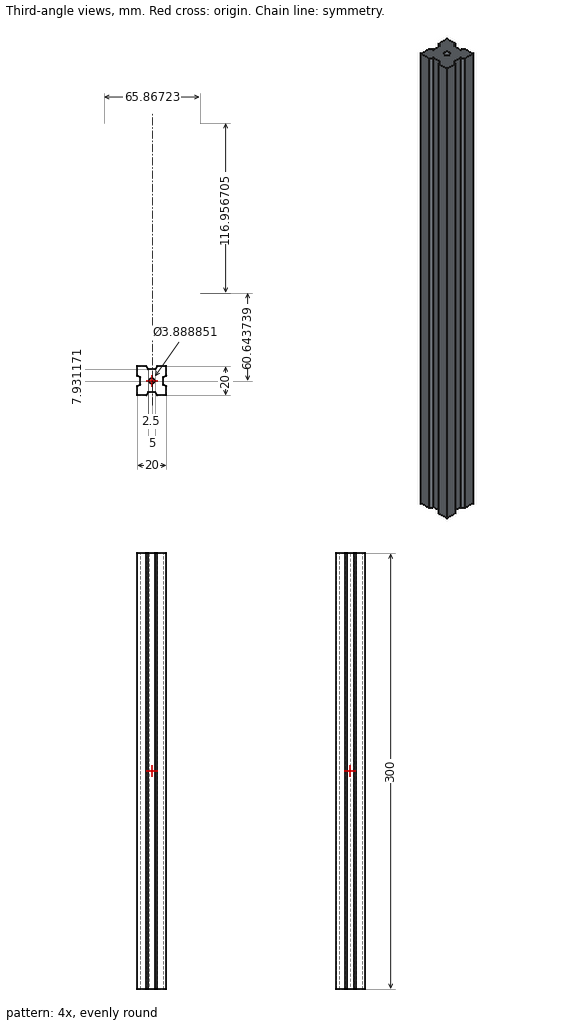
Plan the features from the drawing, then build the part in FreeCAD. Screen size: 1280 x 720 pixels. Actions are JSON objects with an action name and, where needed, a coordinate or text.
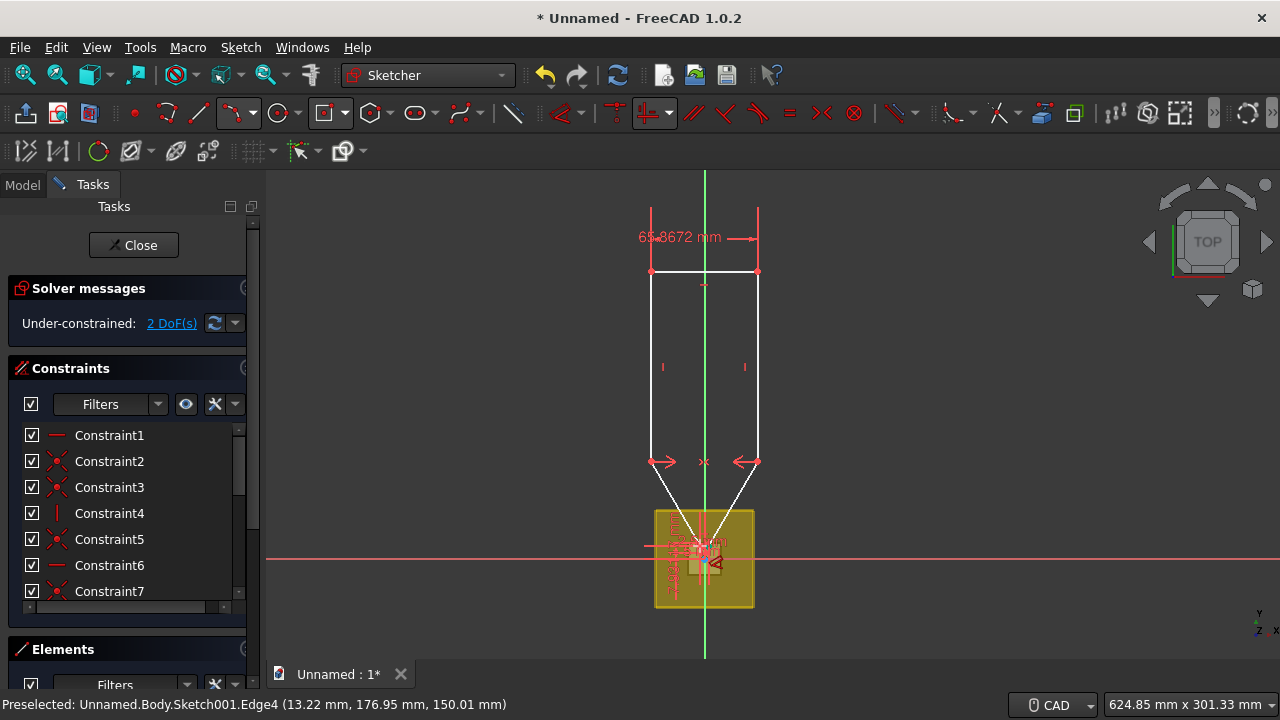
{"action": "left_click", "coordinate": [758, 405]}
{"action": "left_click", "coordinate": [792, 367]}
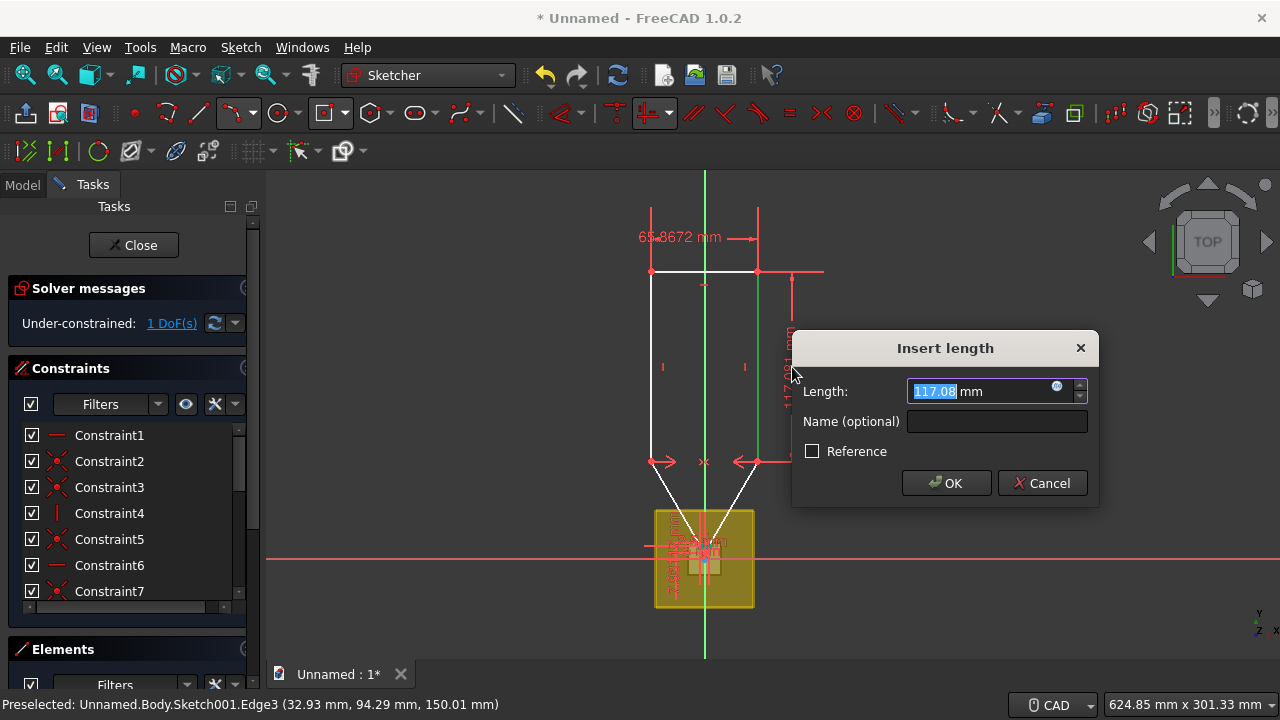
{"action": "type", "text": "116.956705"}
{"action": "key", "text": "Return"}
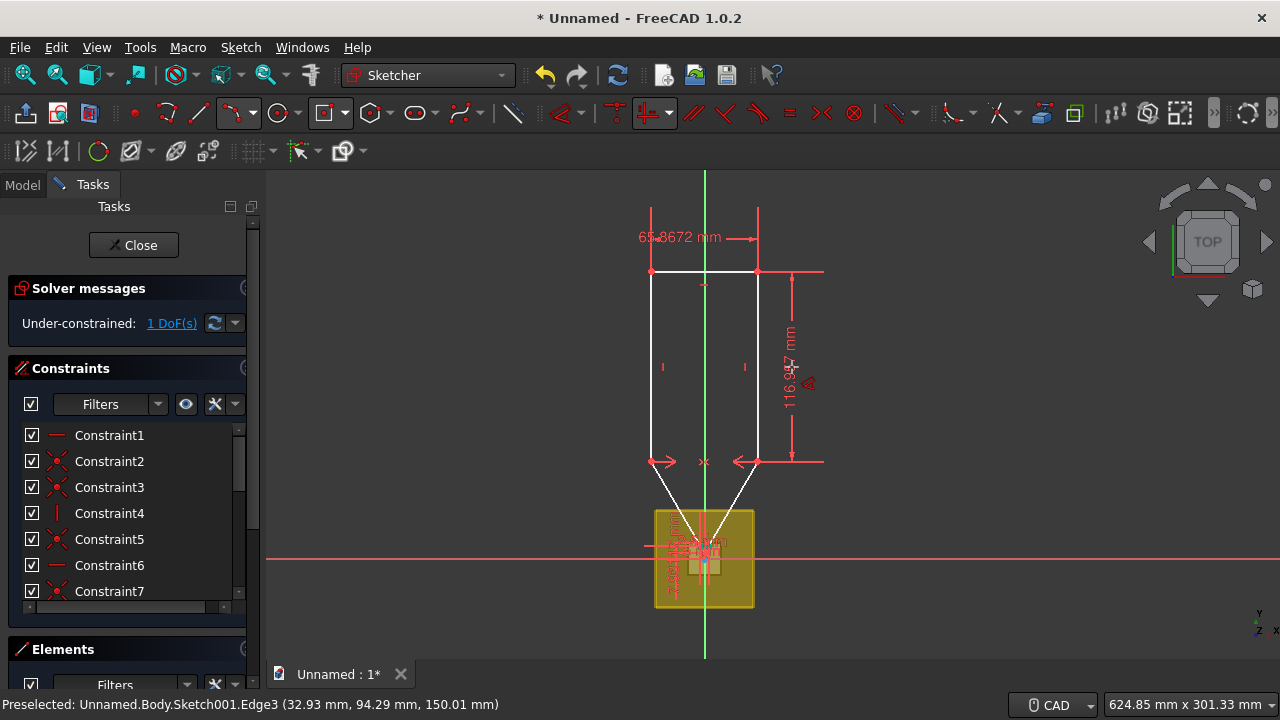
{"action": "left_click", "coordinate": [758, 462]}
{"action": "left_click", "coordinate": [792, 510]}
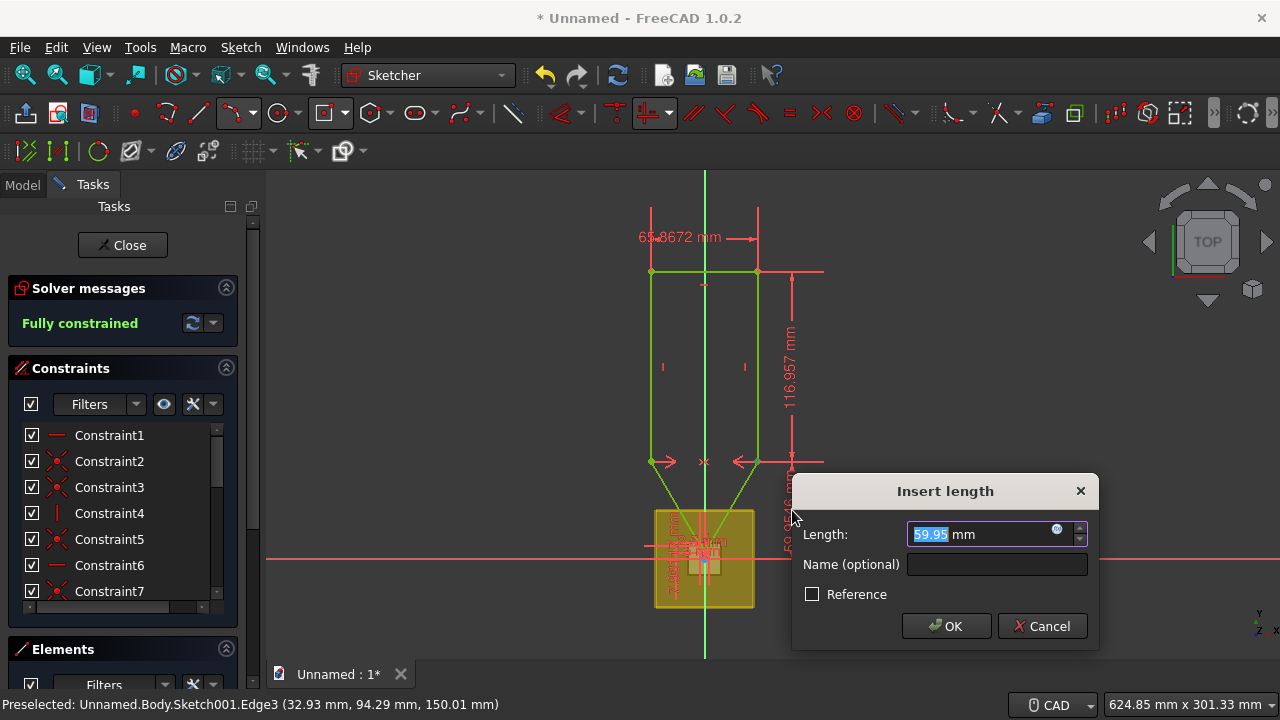
{"action": "type", "text": "60.643739"}
{"action": "key", "text": "Return"}
{"action": "key", "text": "Escape"}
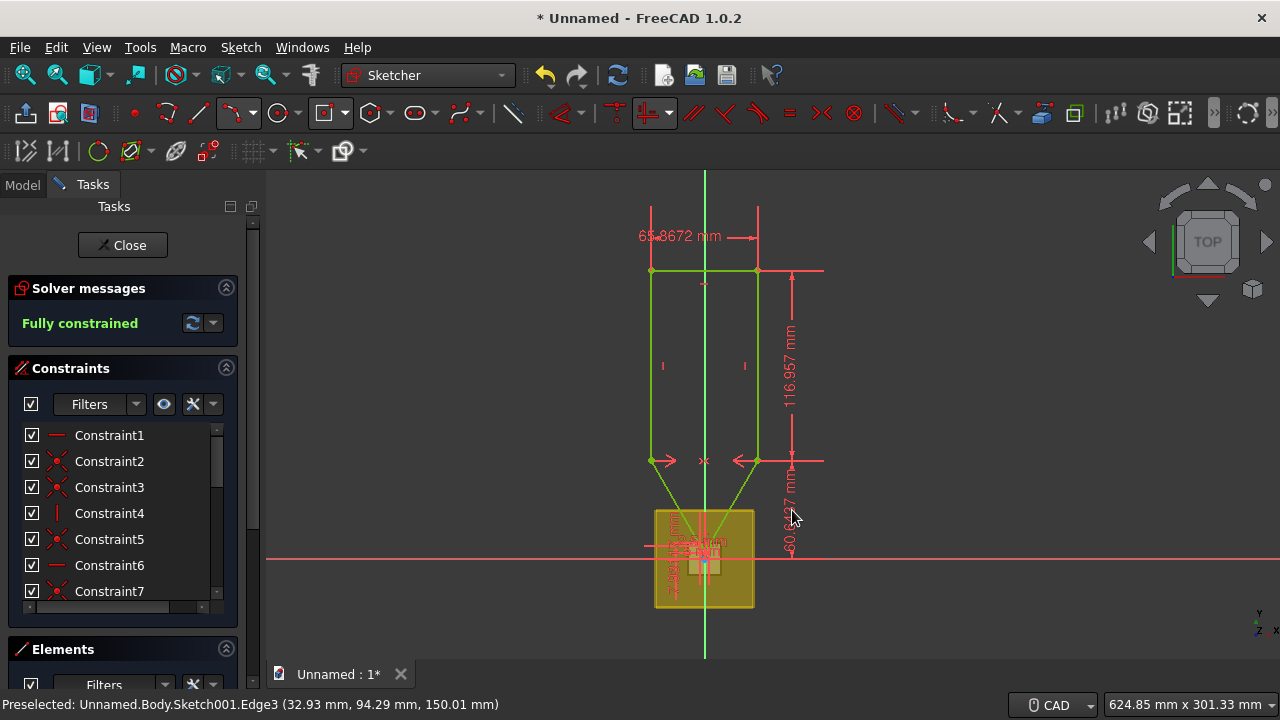
{"action": "left_click", "coordinate": [123, 245]}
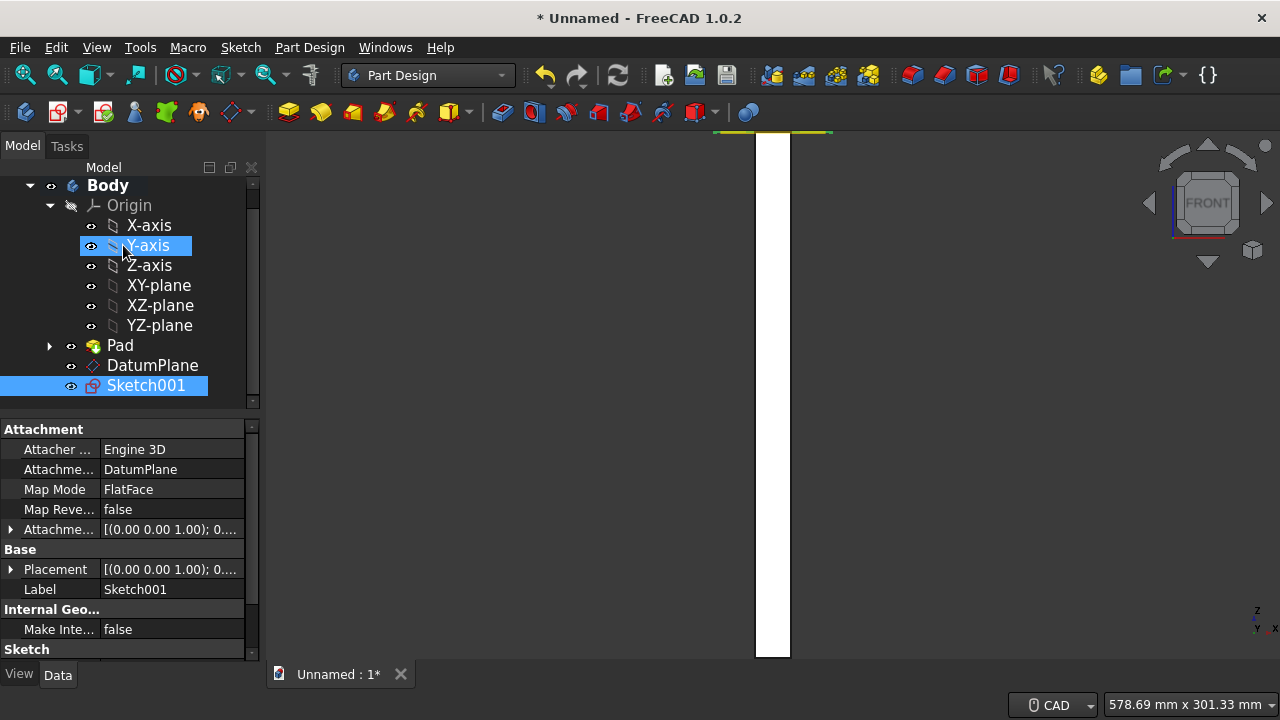
{"action": "left_click", "coordinate": [504, 112]}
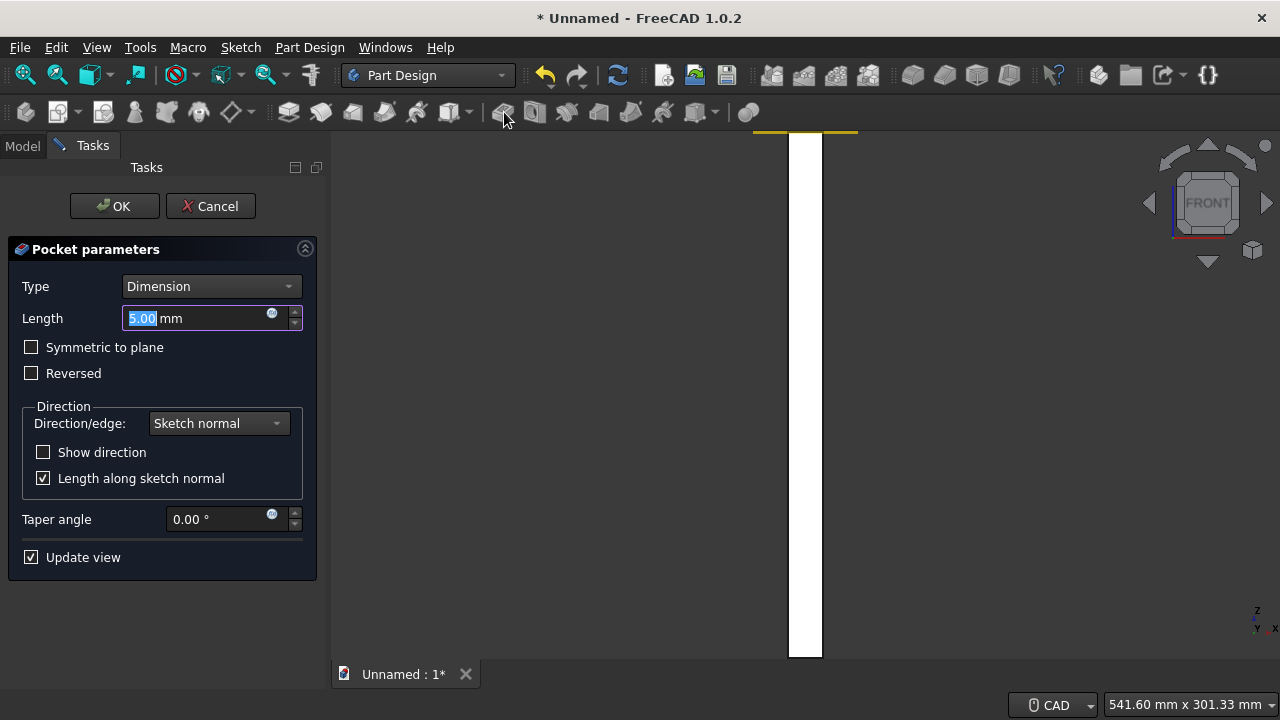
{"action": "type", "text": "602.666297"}
{"action": "key", "text": "Tab"}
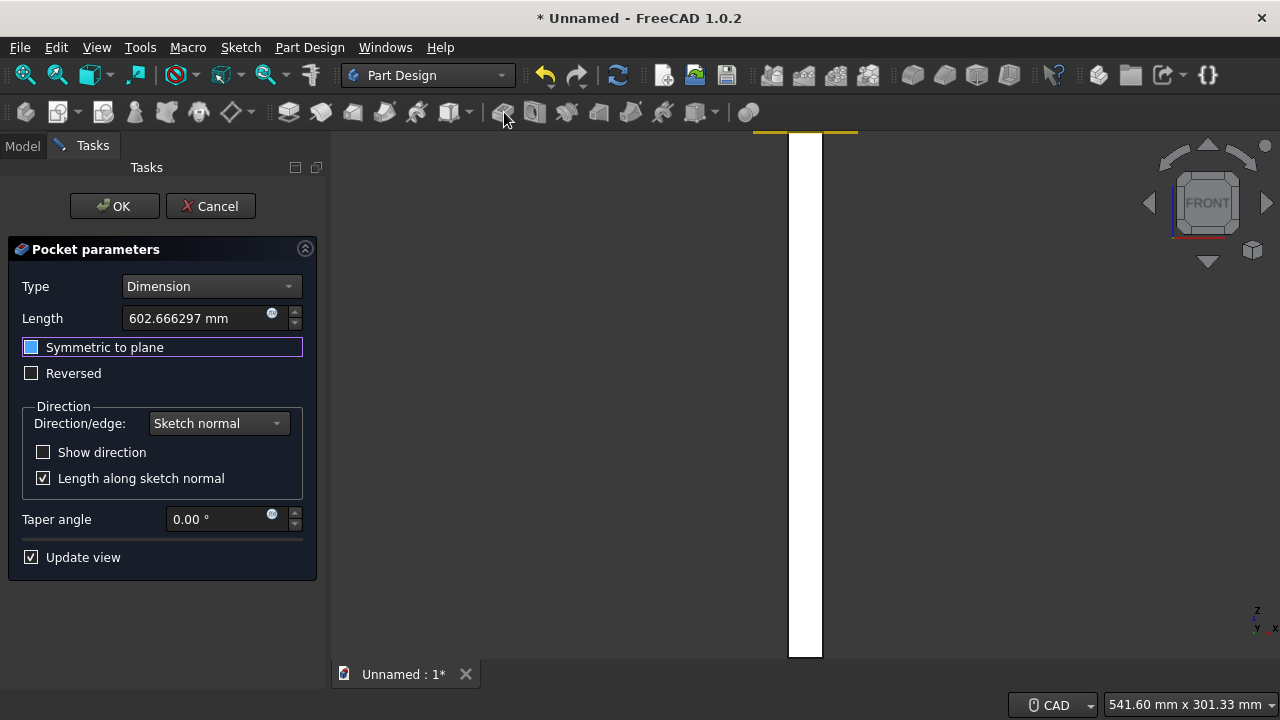
{"action": "left_click", "coordinate": [30, 347]}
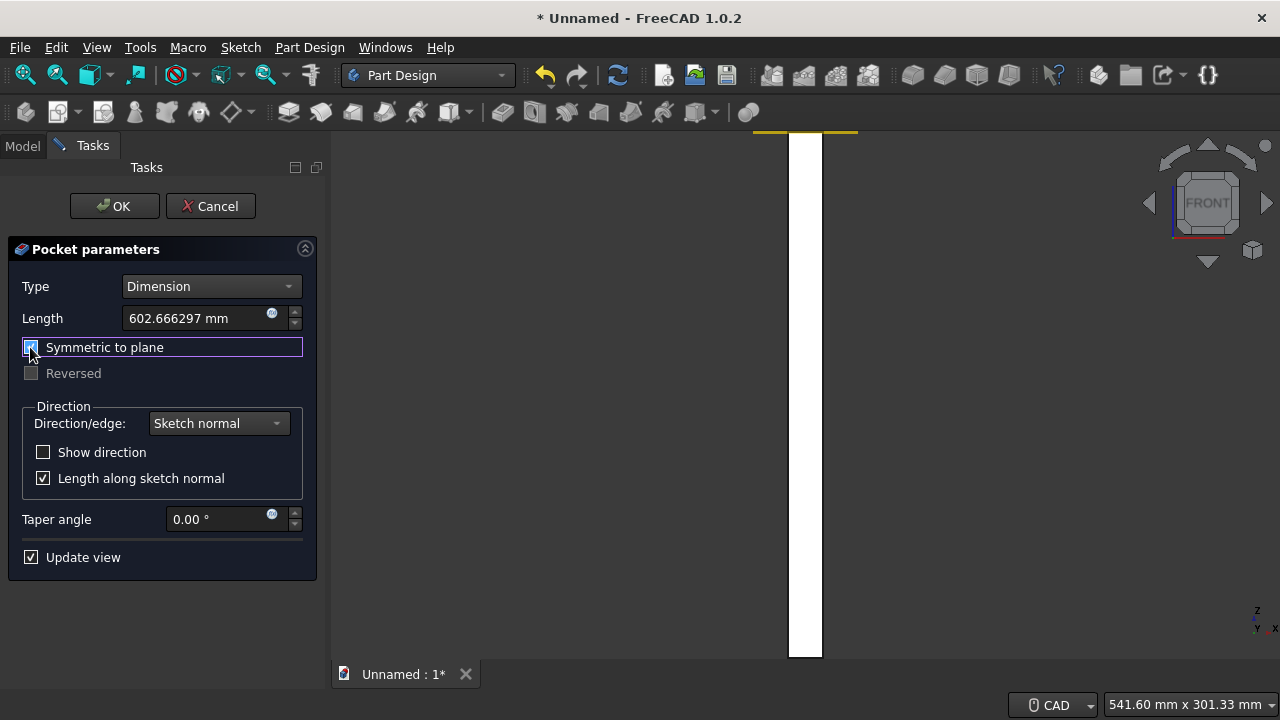
{"action": "left_click", "coordinate": [115, 206]}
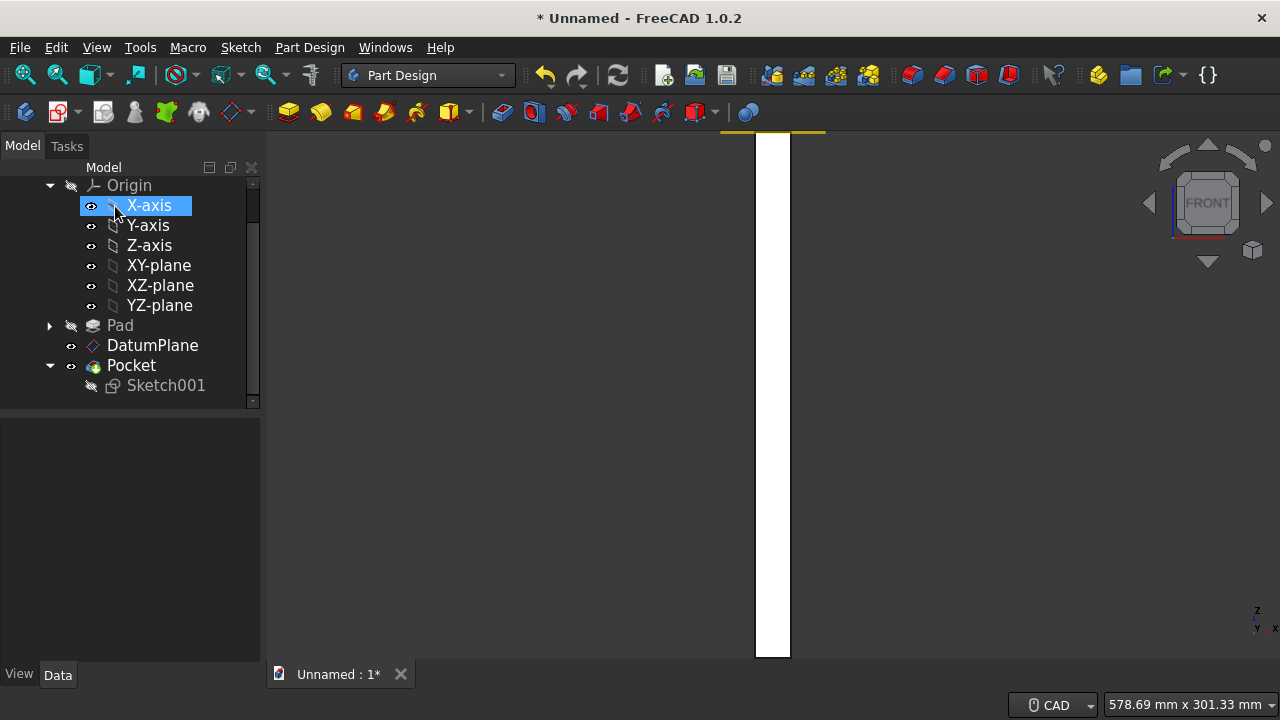
{"action": "left_click", "coordinate": [116, 346]}
{"action": "key", "text": "space"}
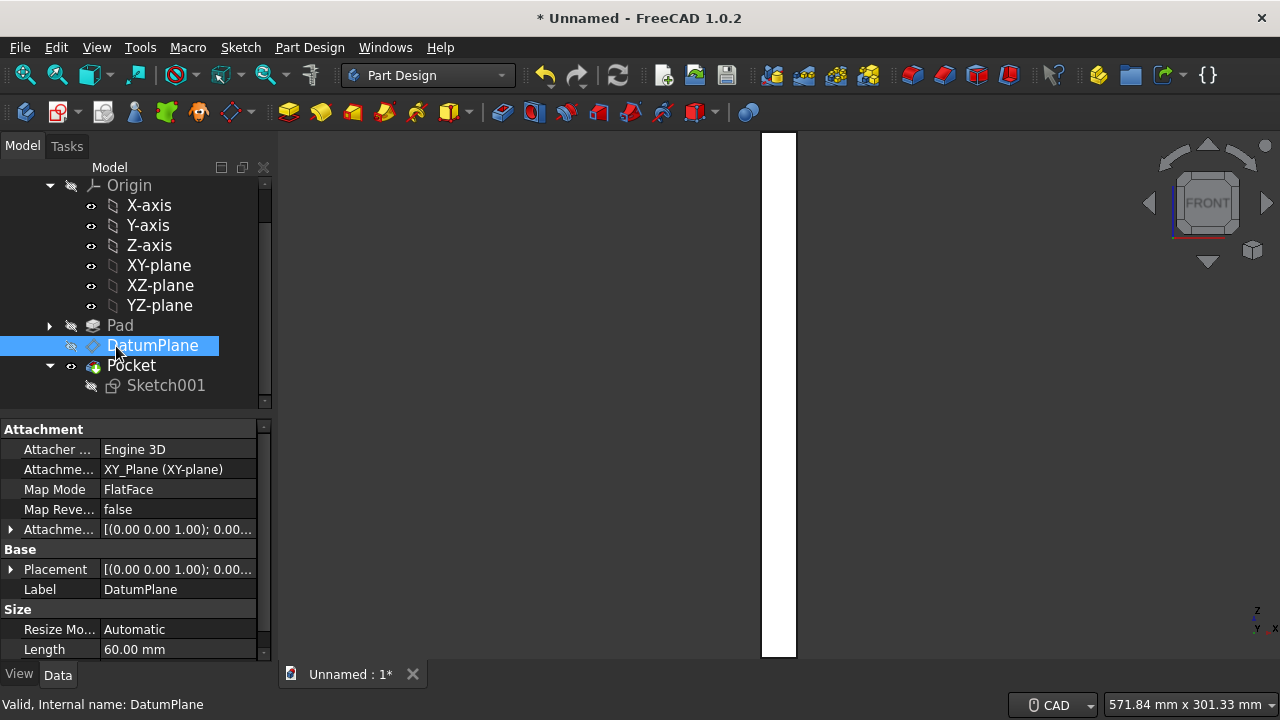
{"action": "left_click", "coordinate": [116, 366]}